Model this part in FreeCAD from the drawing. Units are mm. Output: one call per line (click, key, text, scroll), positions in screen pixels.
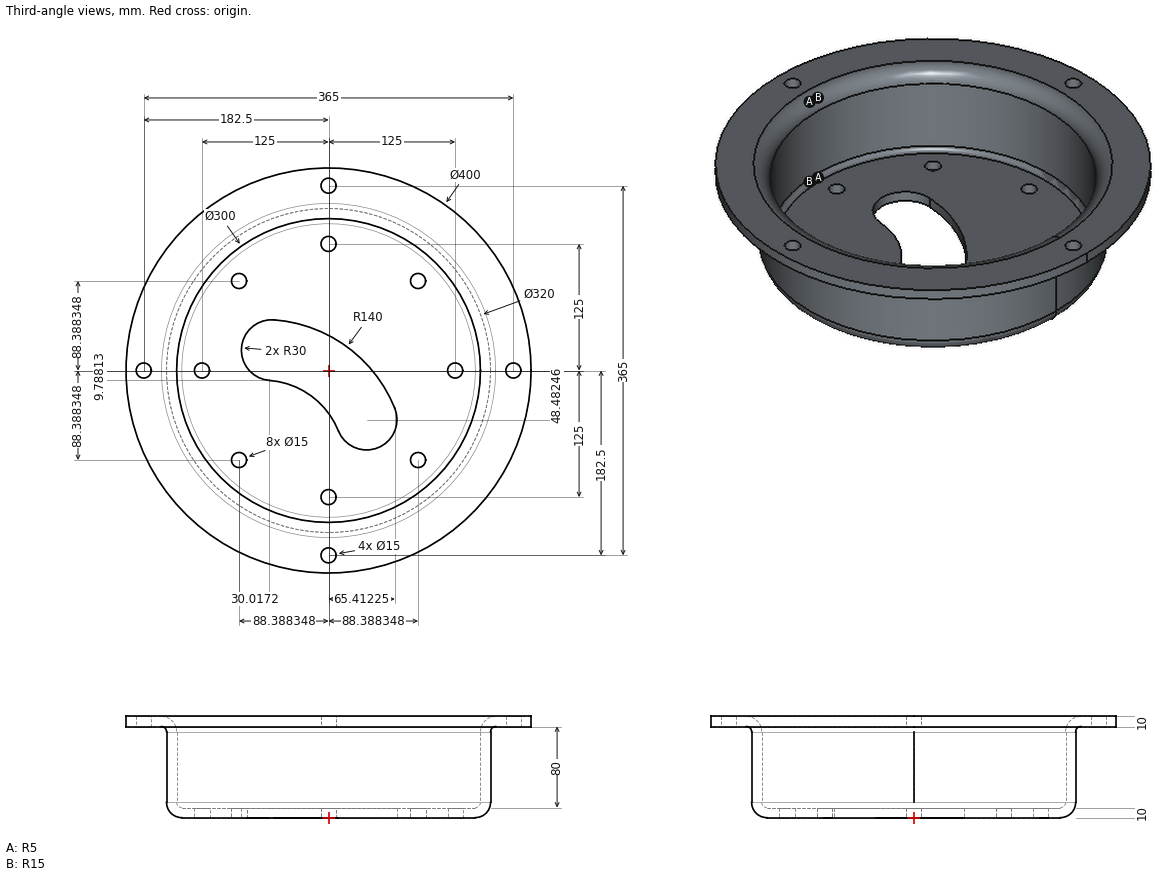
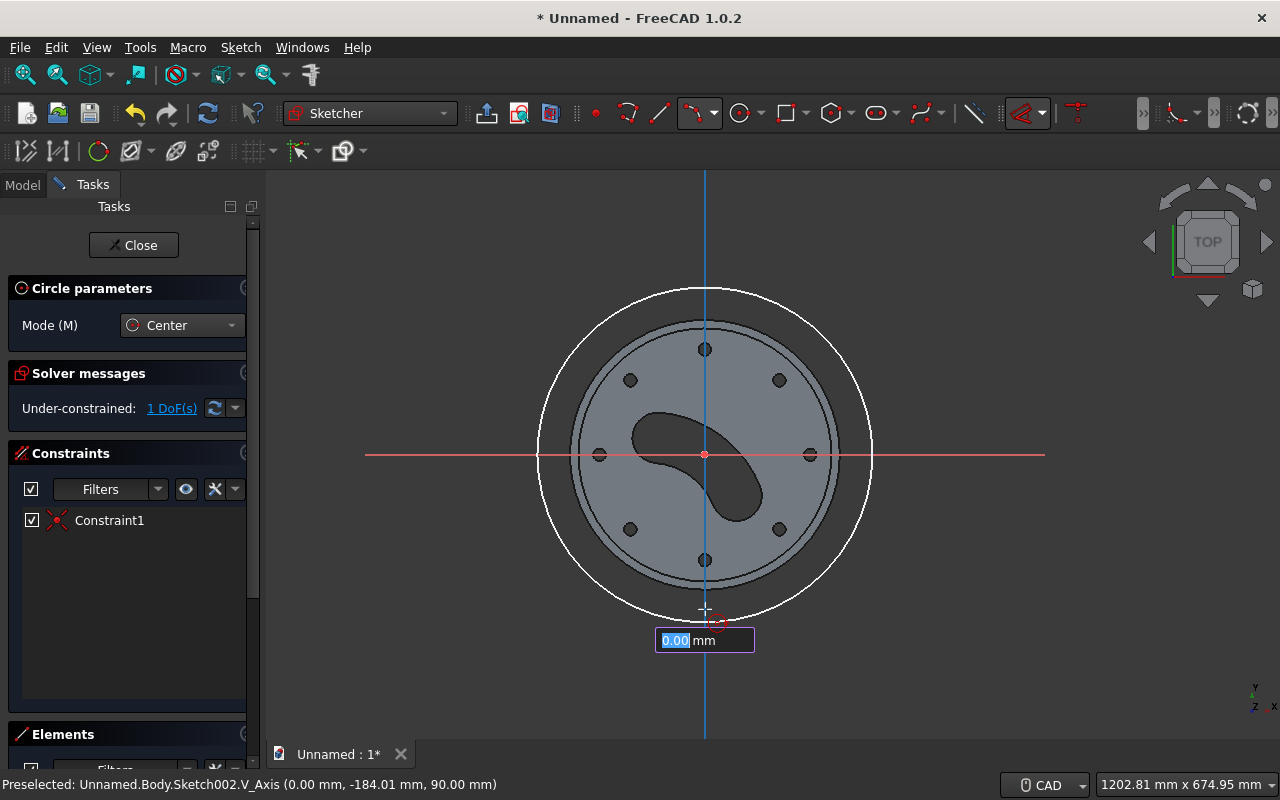
scroll(711, 607, up, 5)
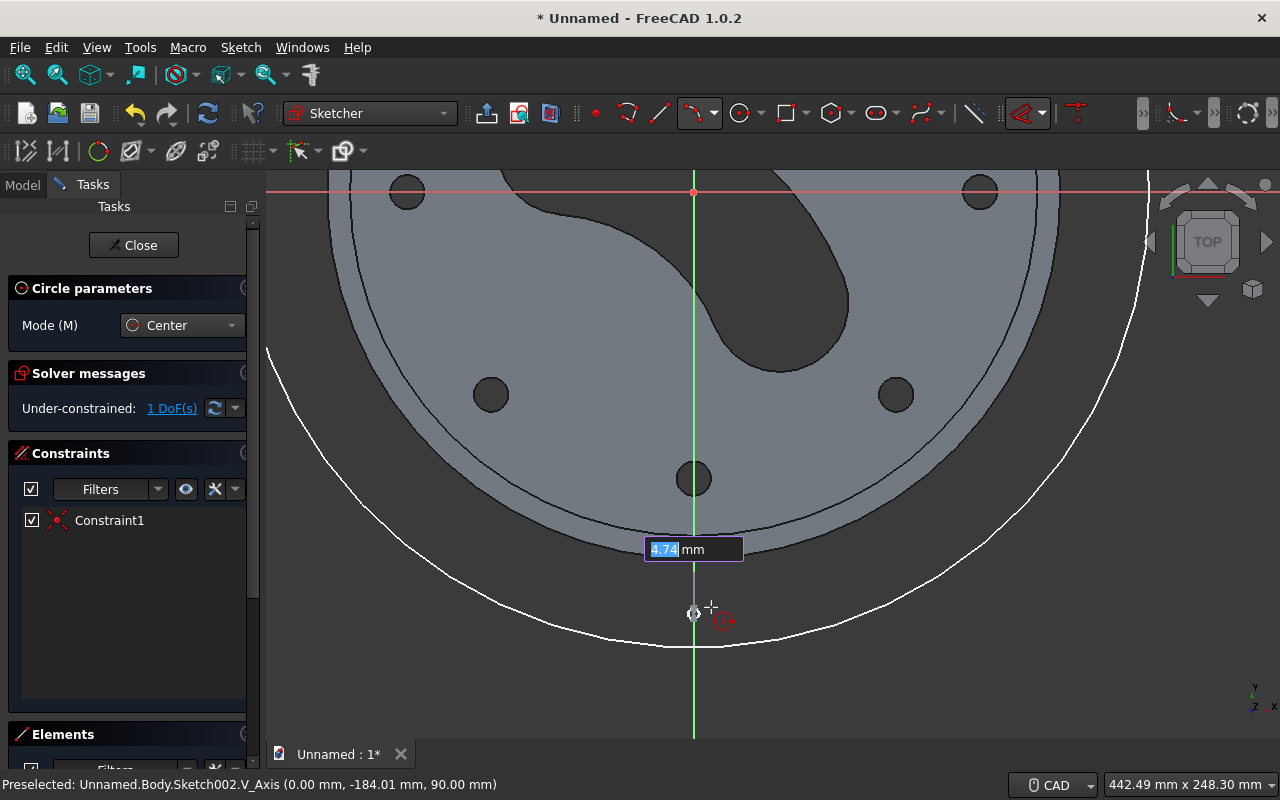
click(710, 604)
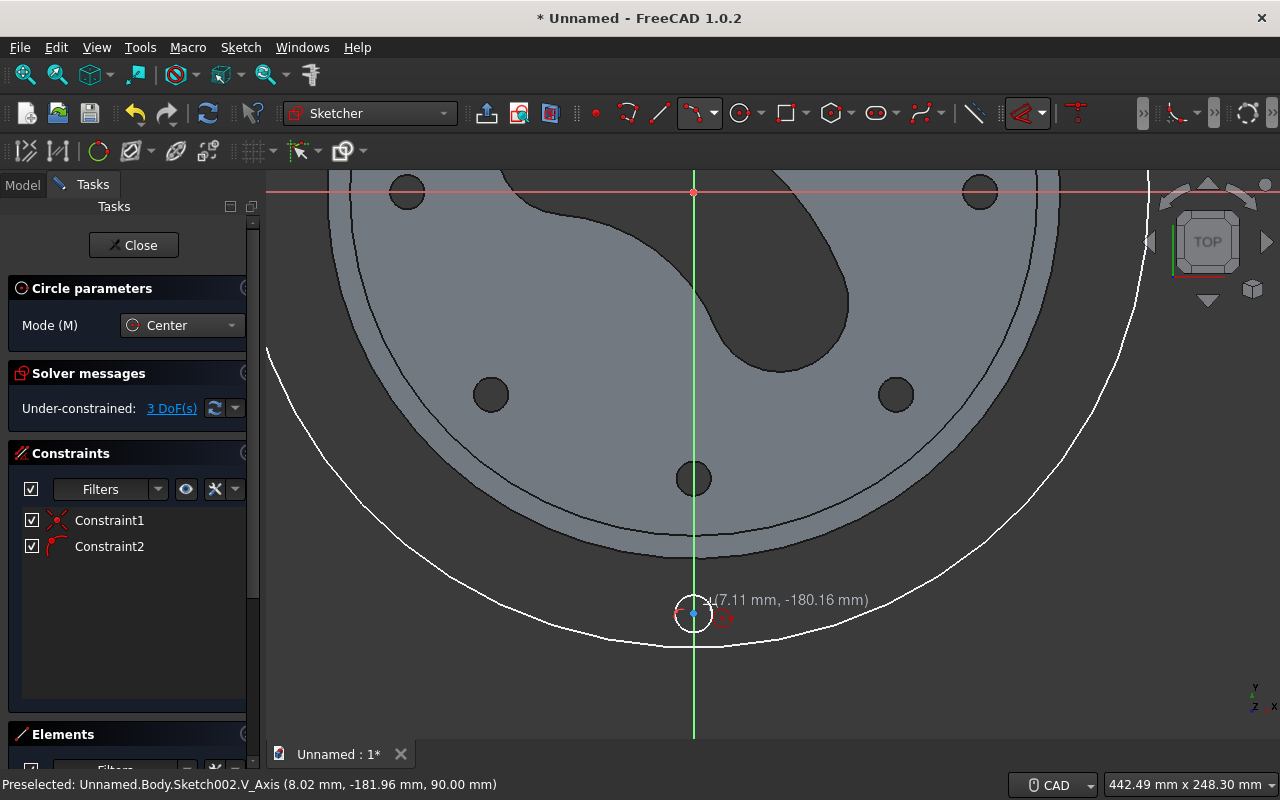
scroll(711, 607, down, 5)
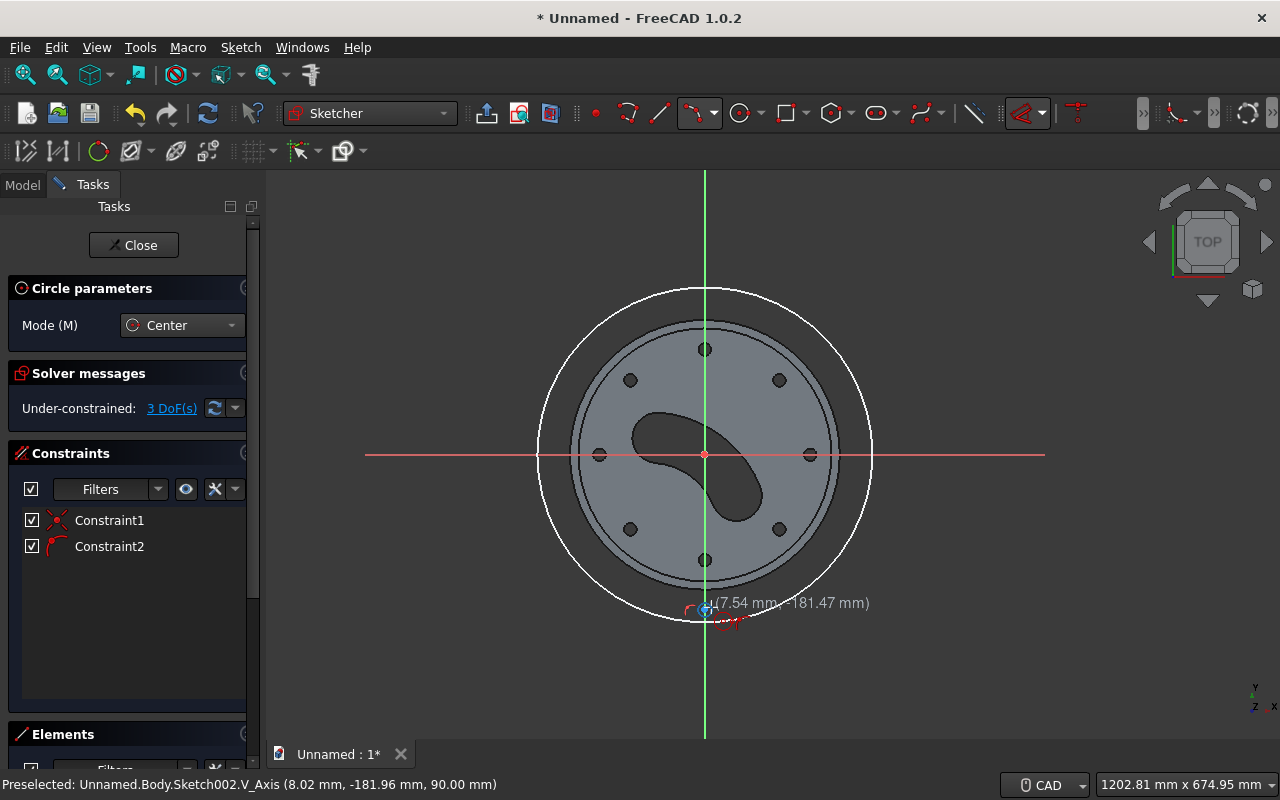
scroll(551, 455, up, 7)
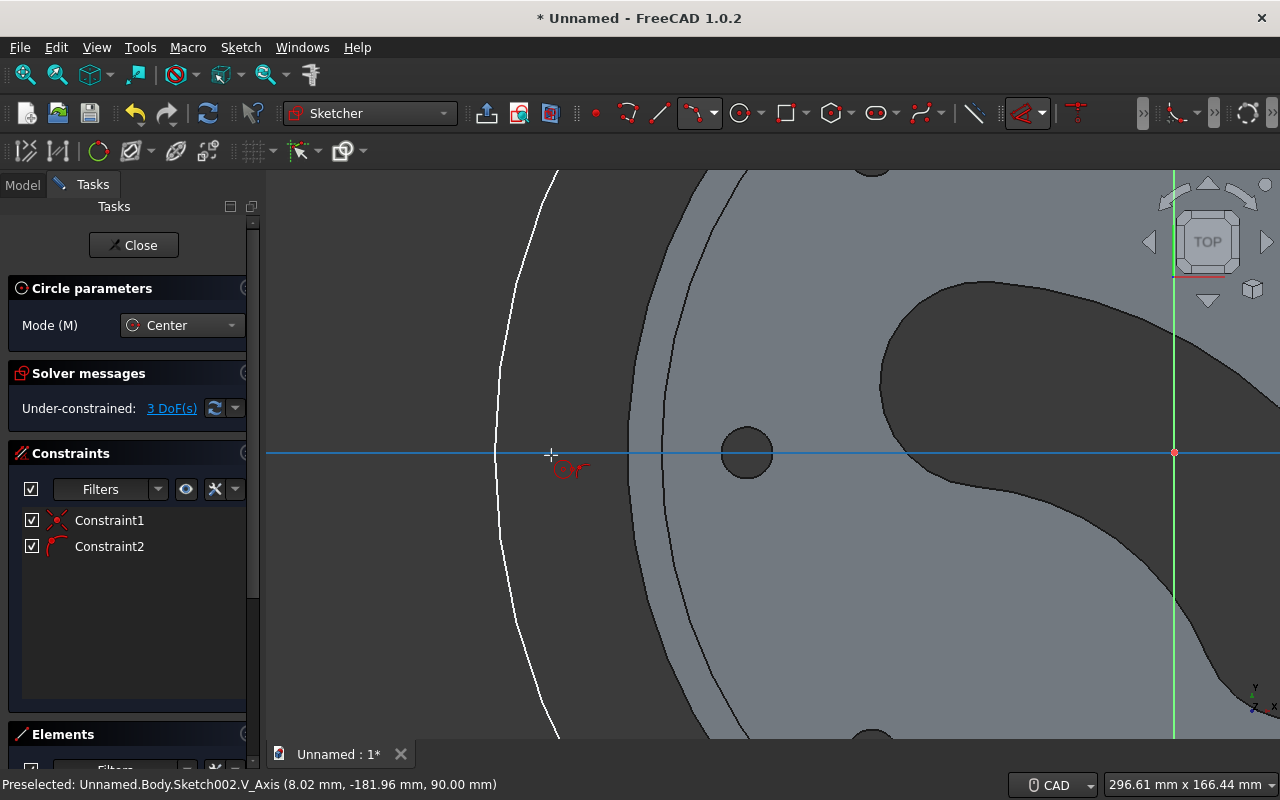
scroll(551, 455, down, 7)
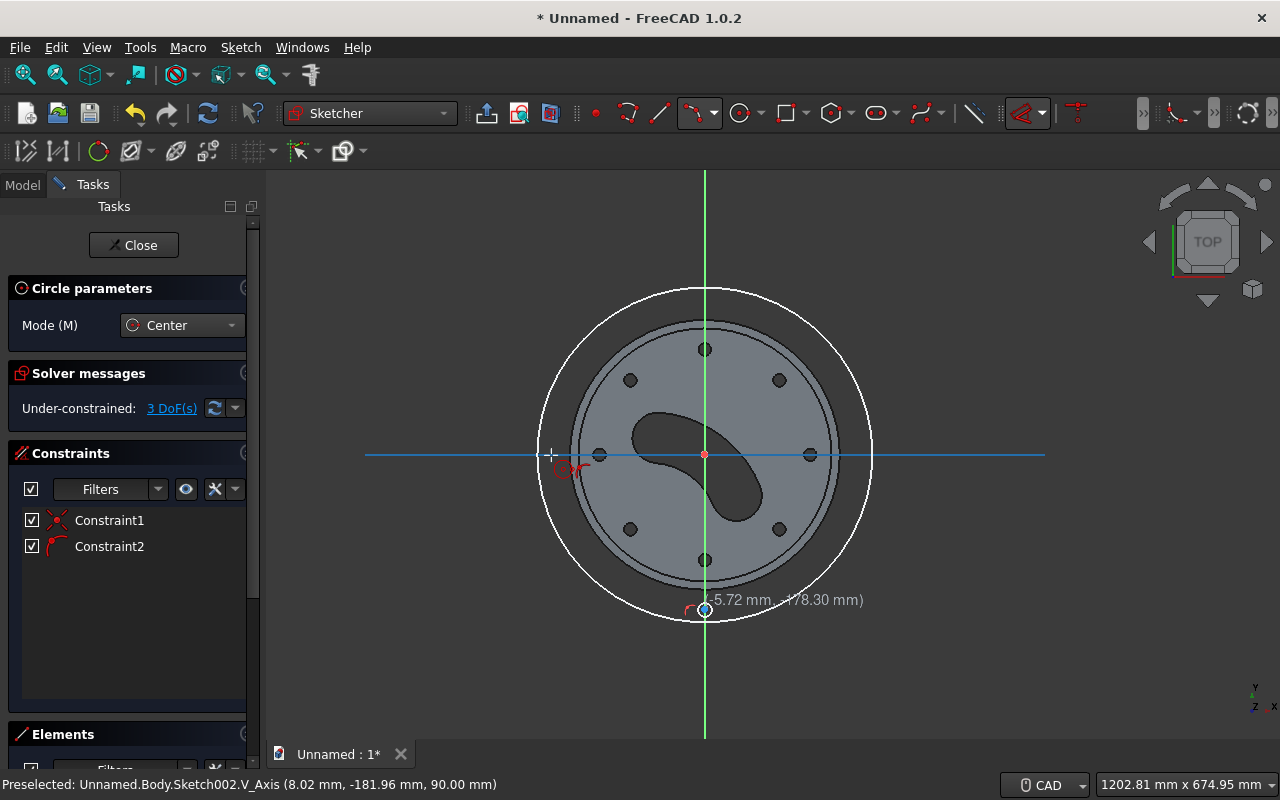
click(551, 455)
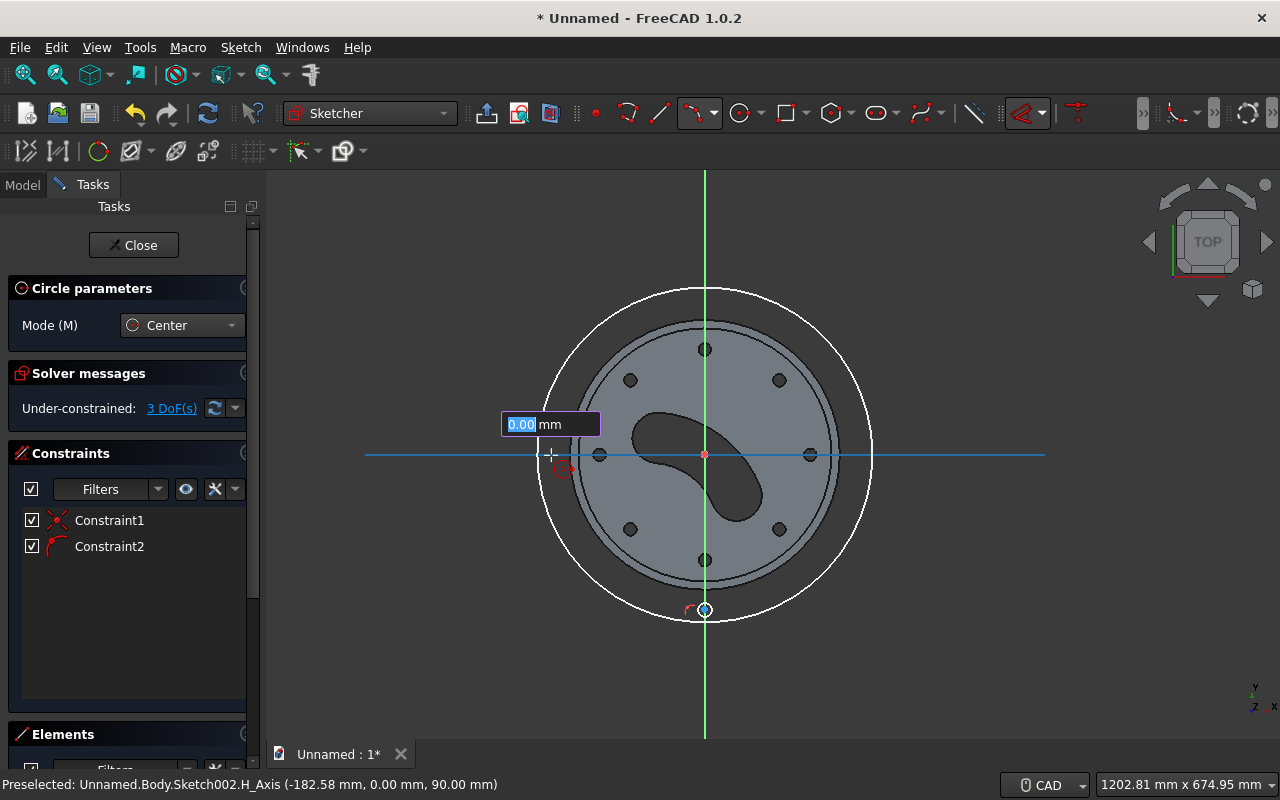
scroll(549, 461, up, 5)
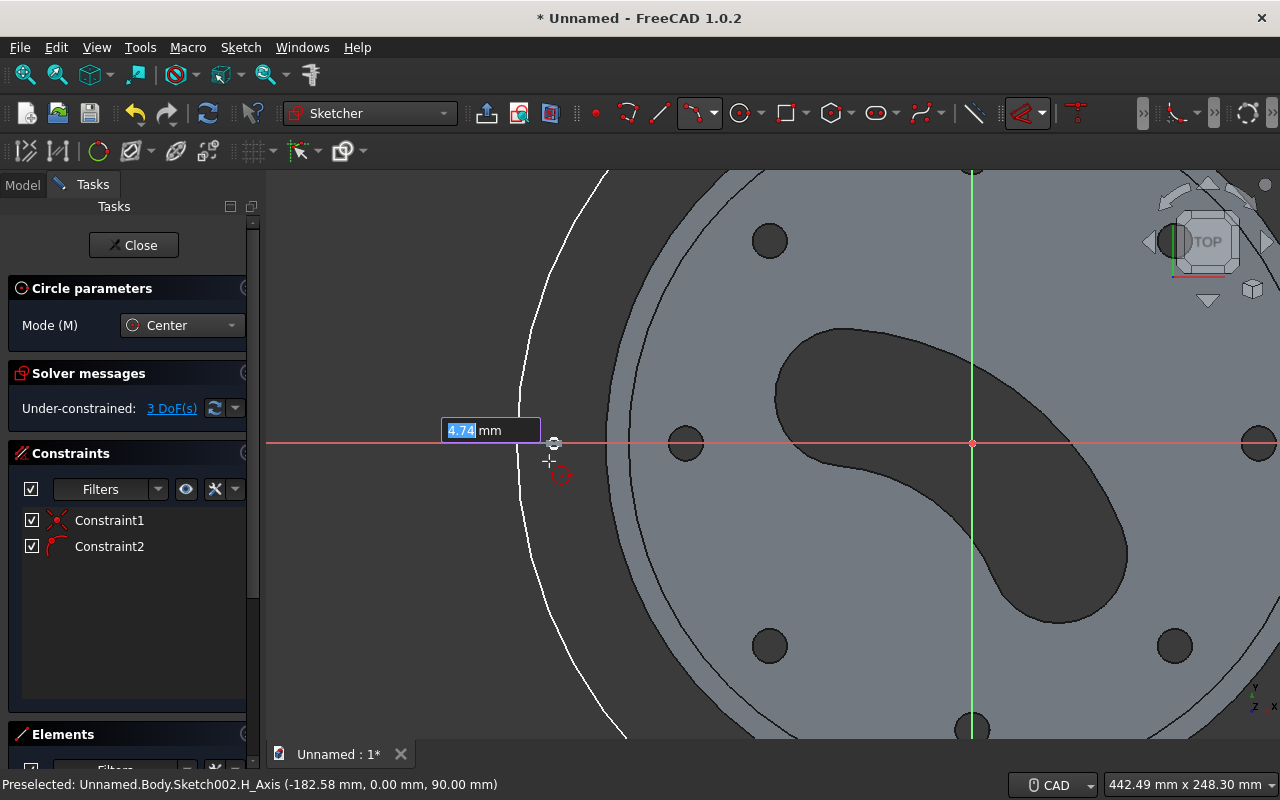
click(548, 460)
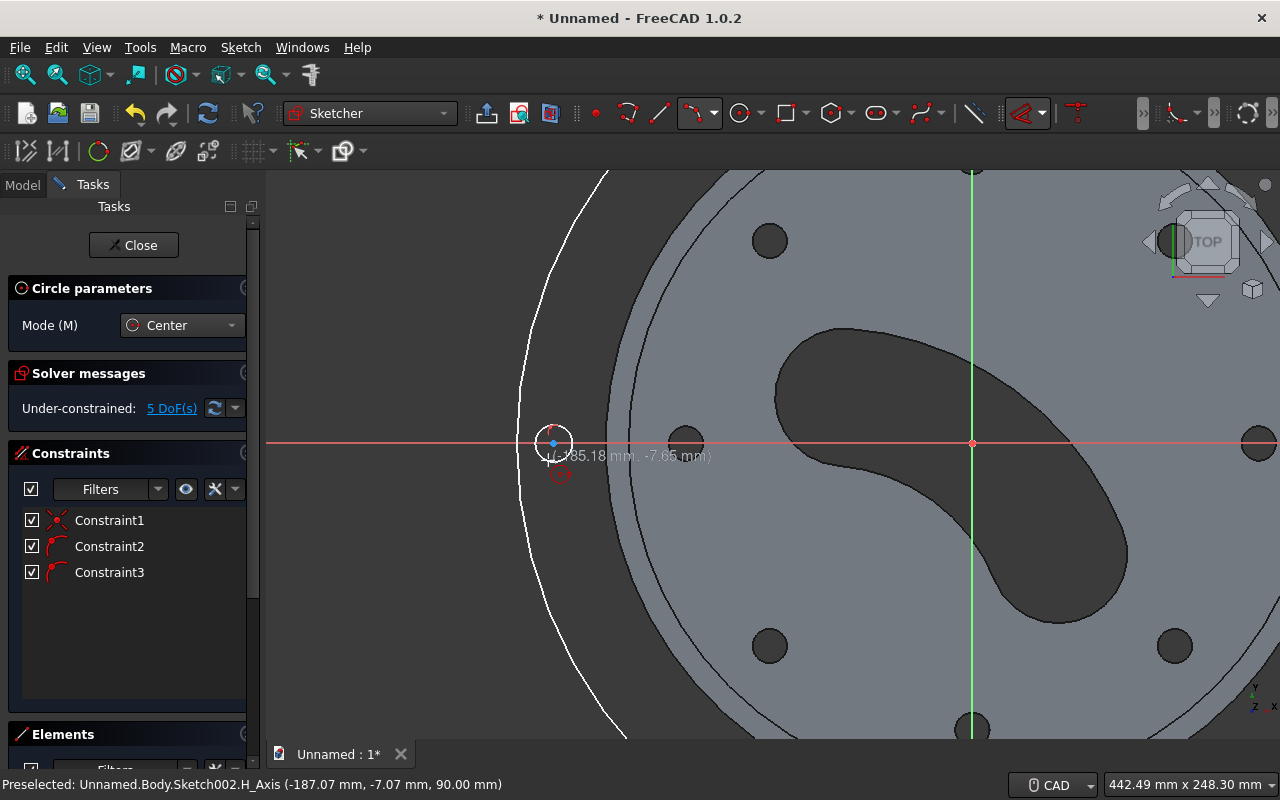
click(972, 443)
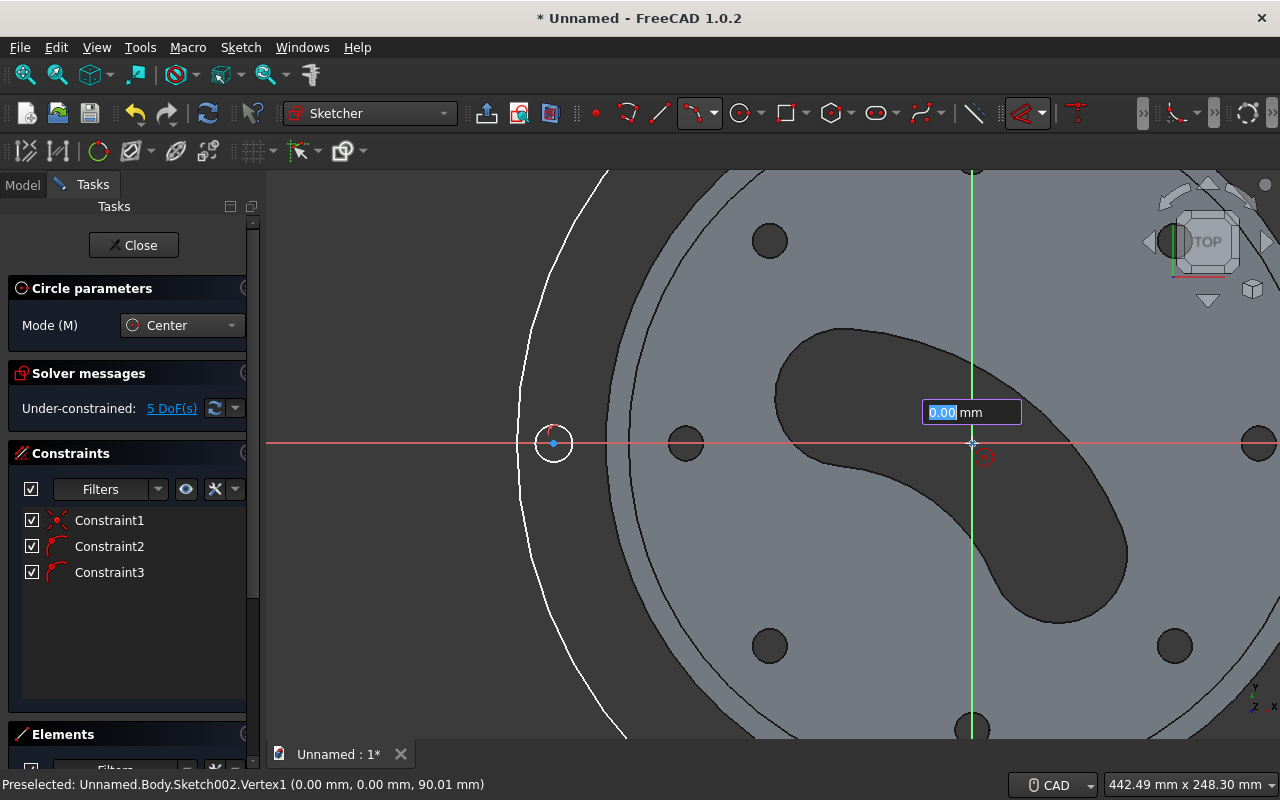
scroll(549, 461, down, 5)